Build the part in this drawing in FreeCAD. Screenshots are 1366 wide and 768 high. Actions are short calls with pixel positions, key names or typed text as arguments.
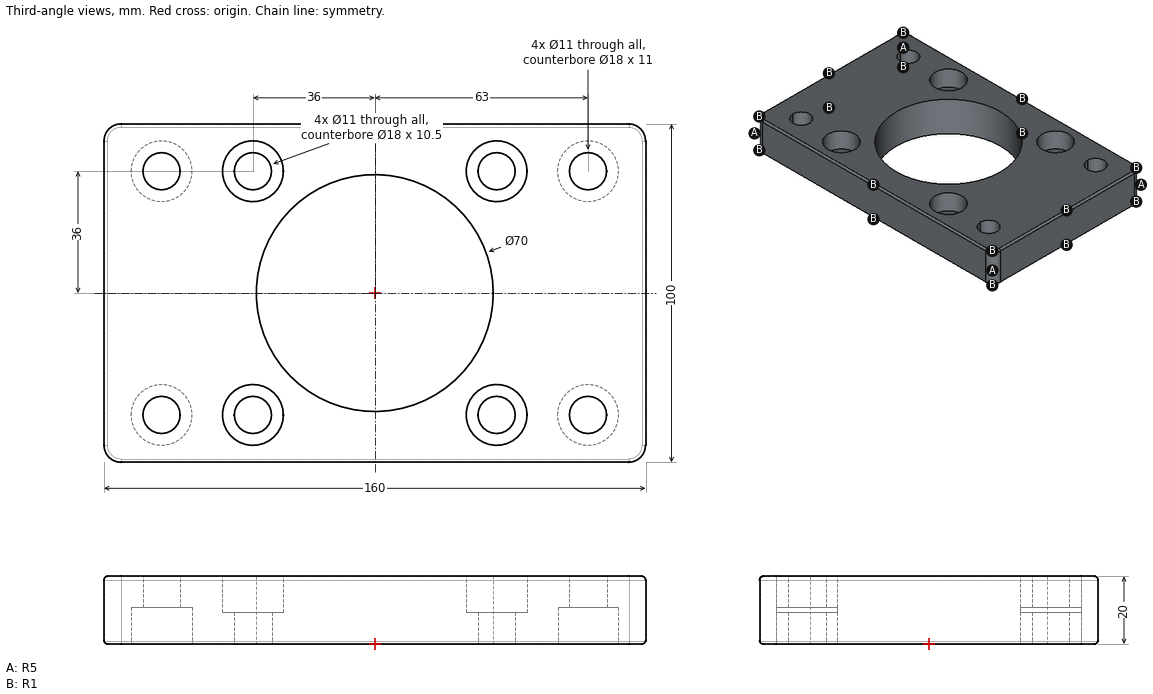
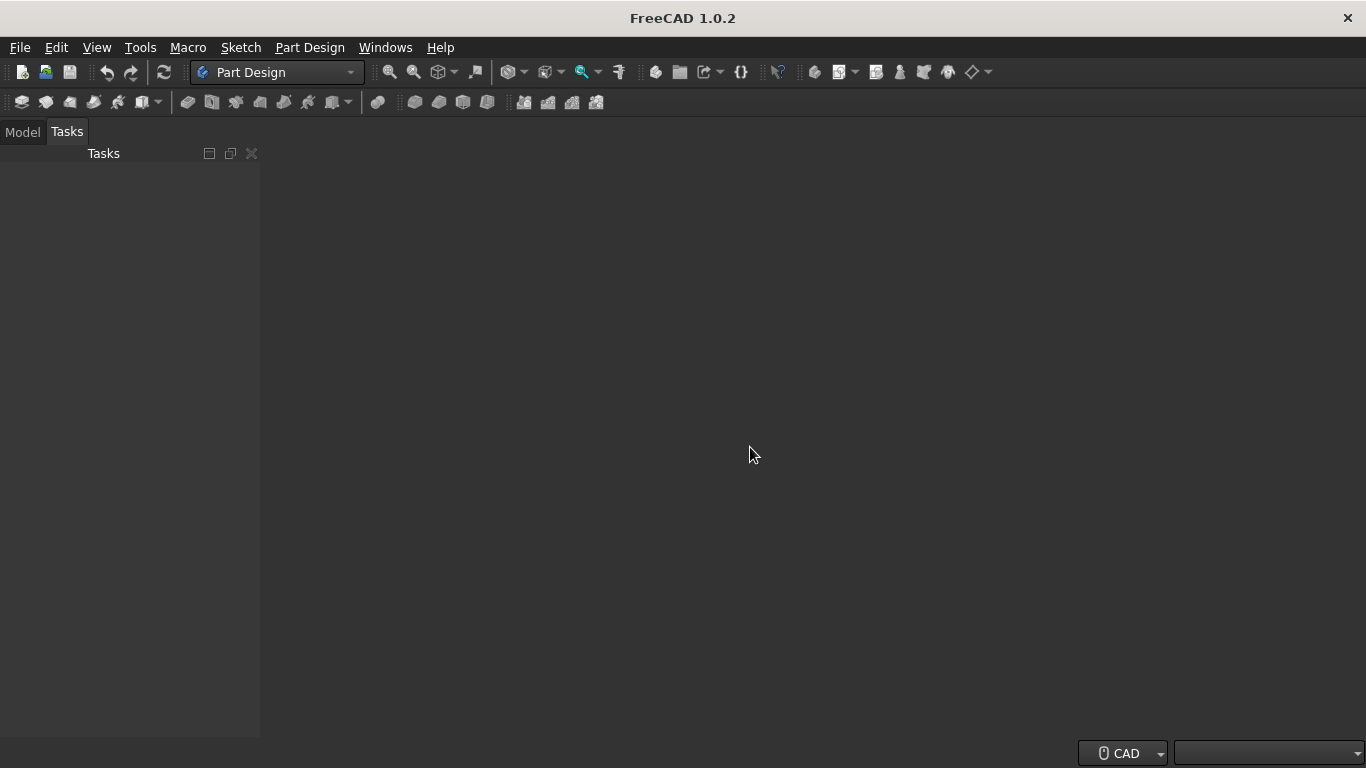
key(ctrl+n)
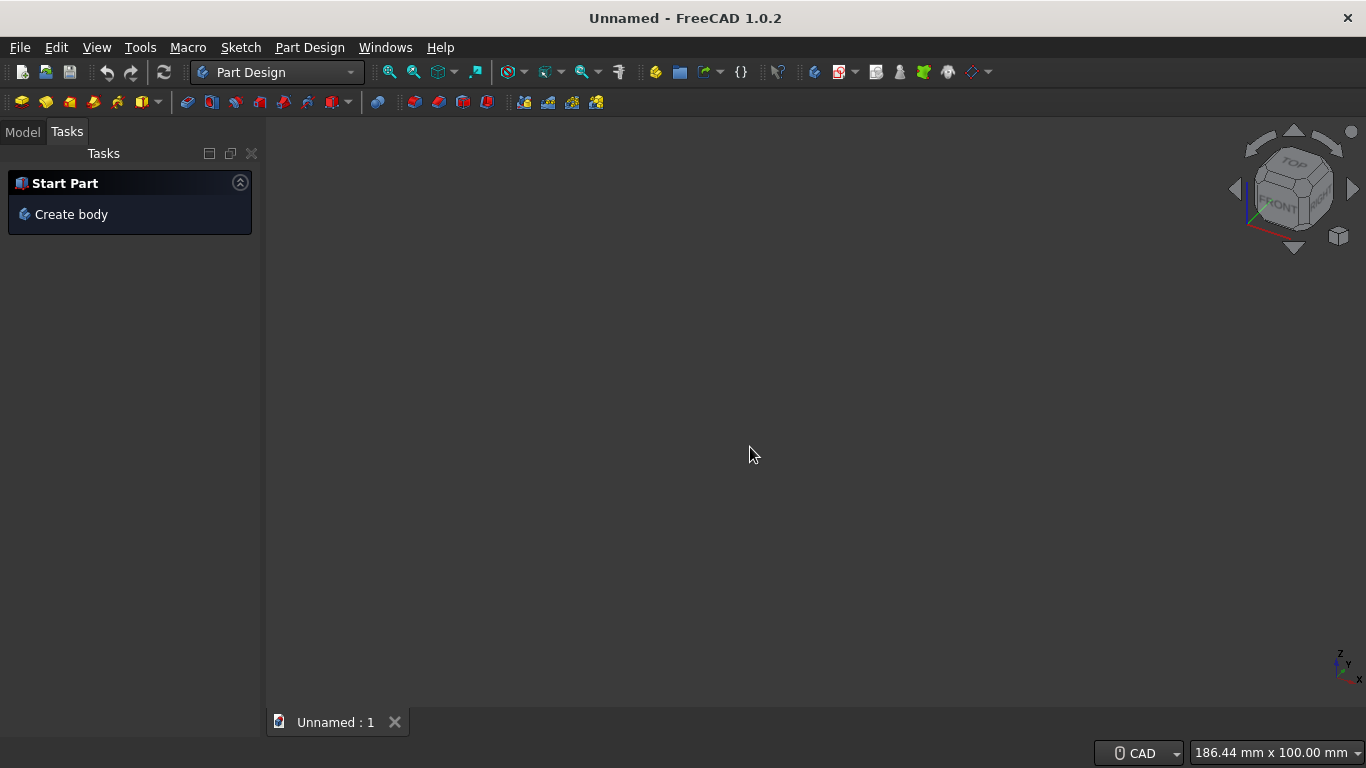
click(840, 72)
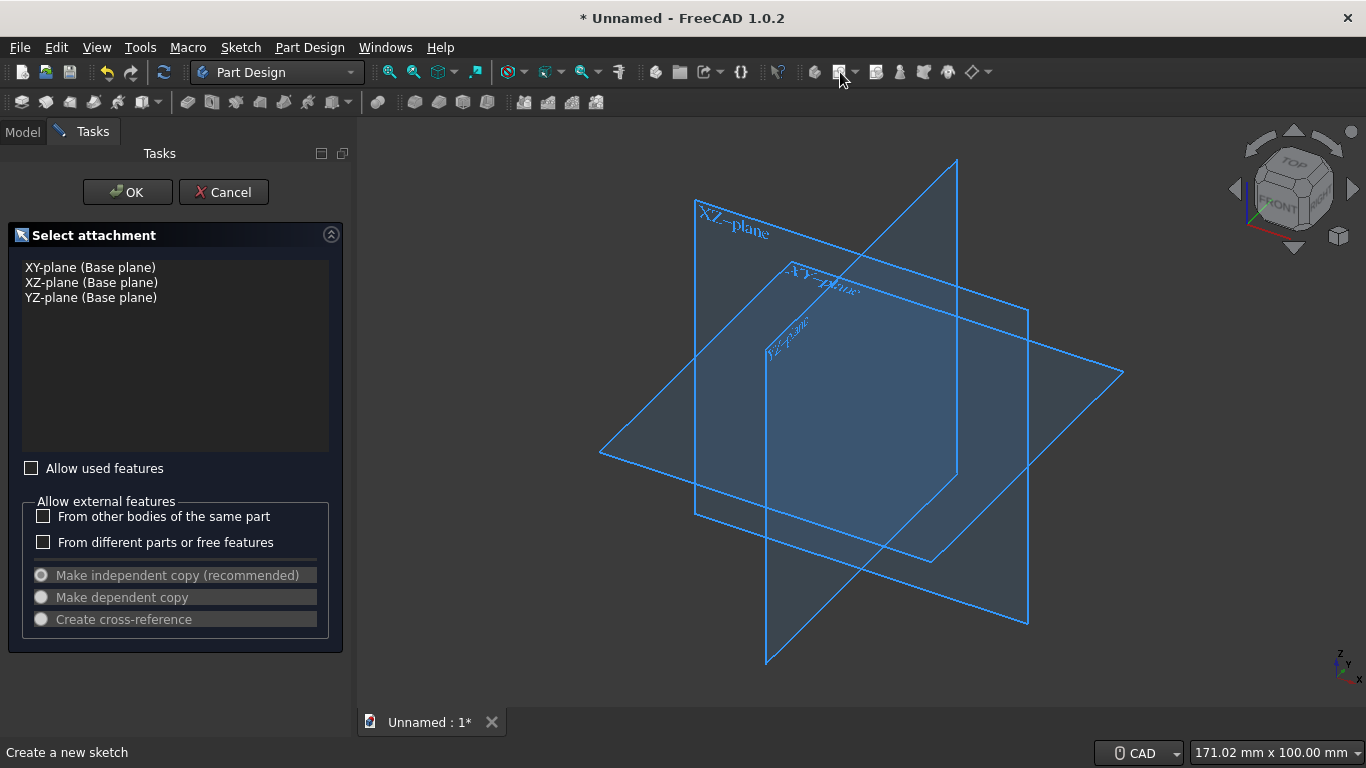
click(82, 268)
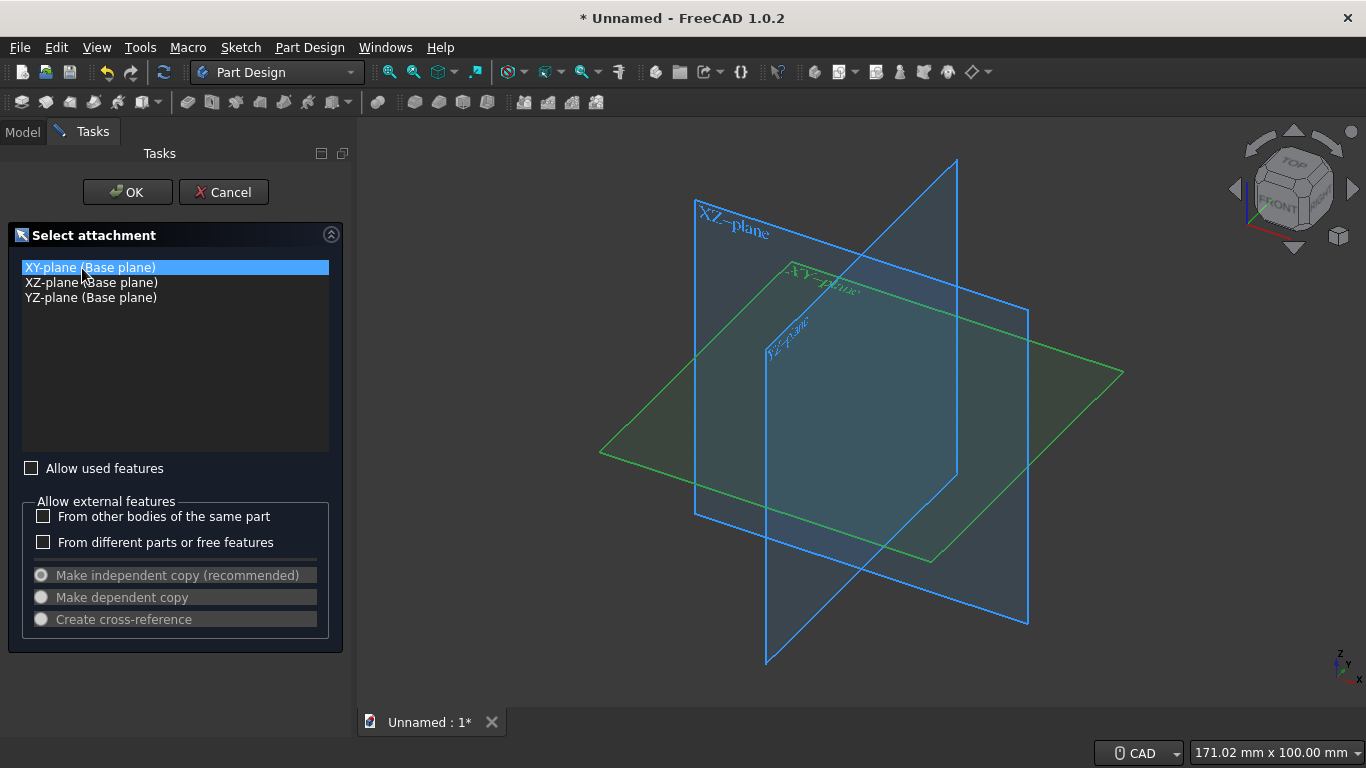
click(128, 192)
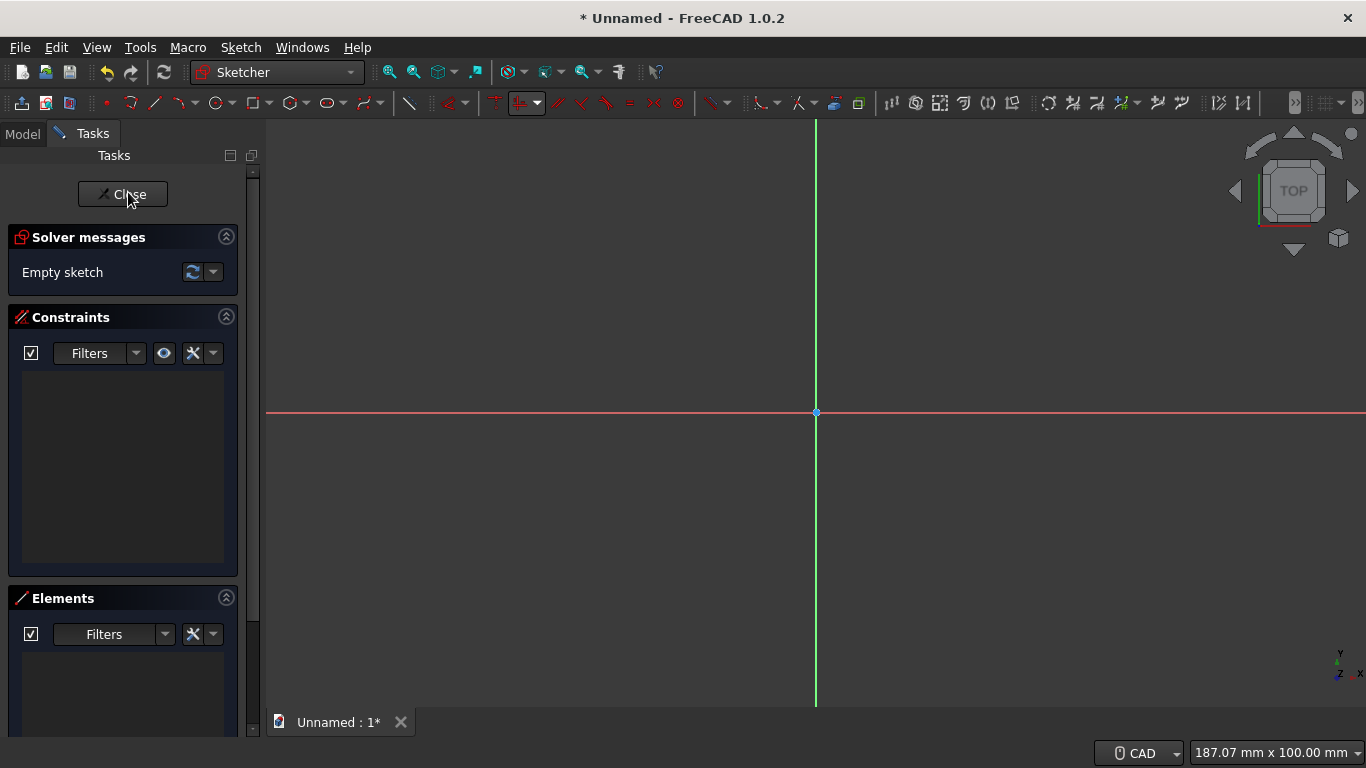
scroll(608, 413, down, 2)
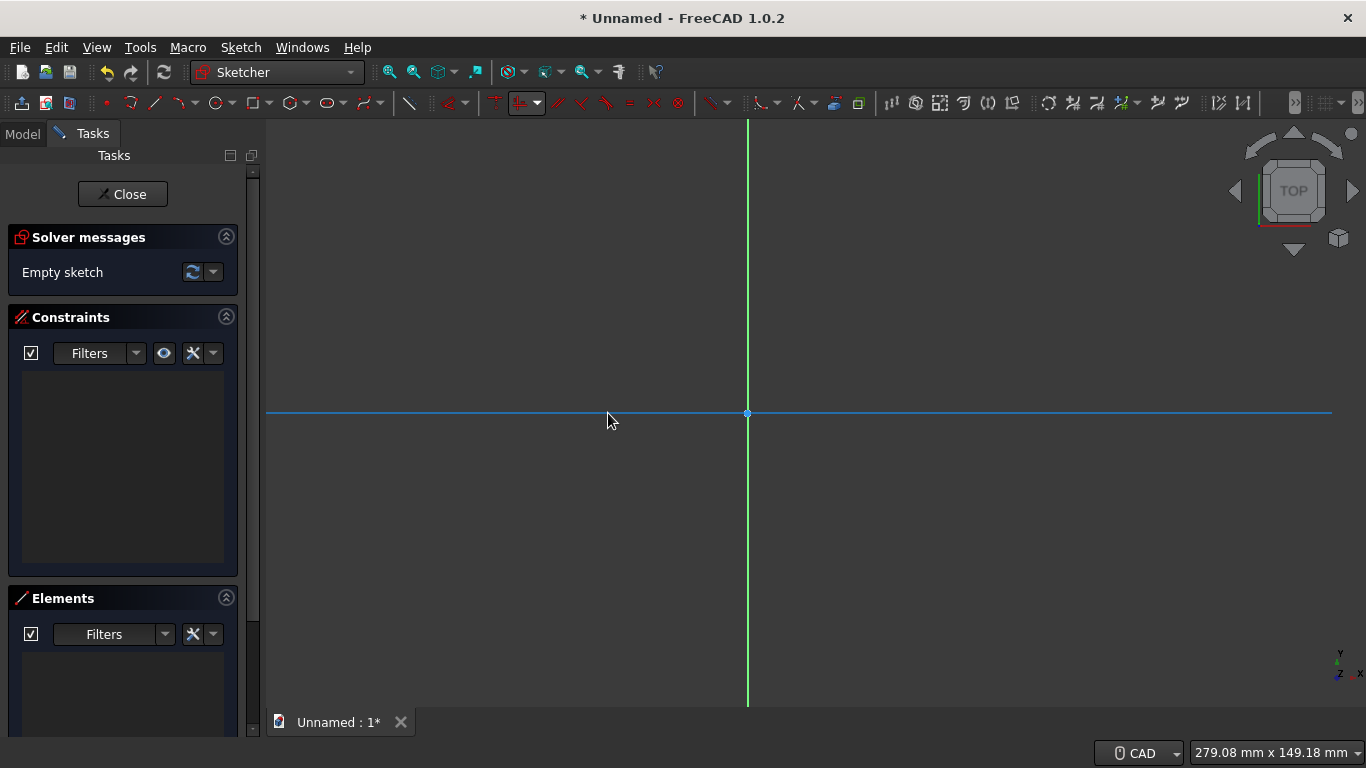
key(g)
key(v)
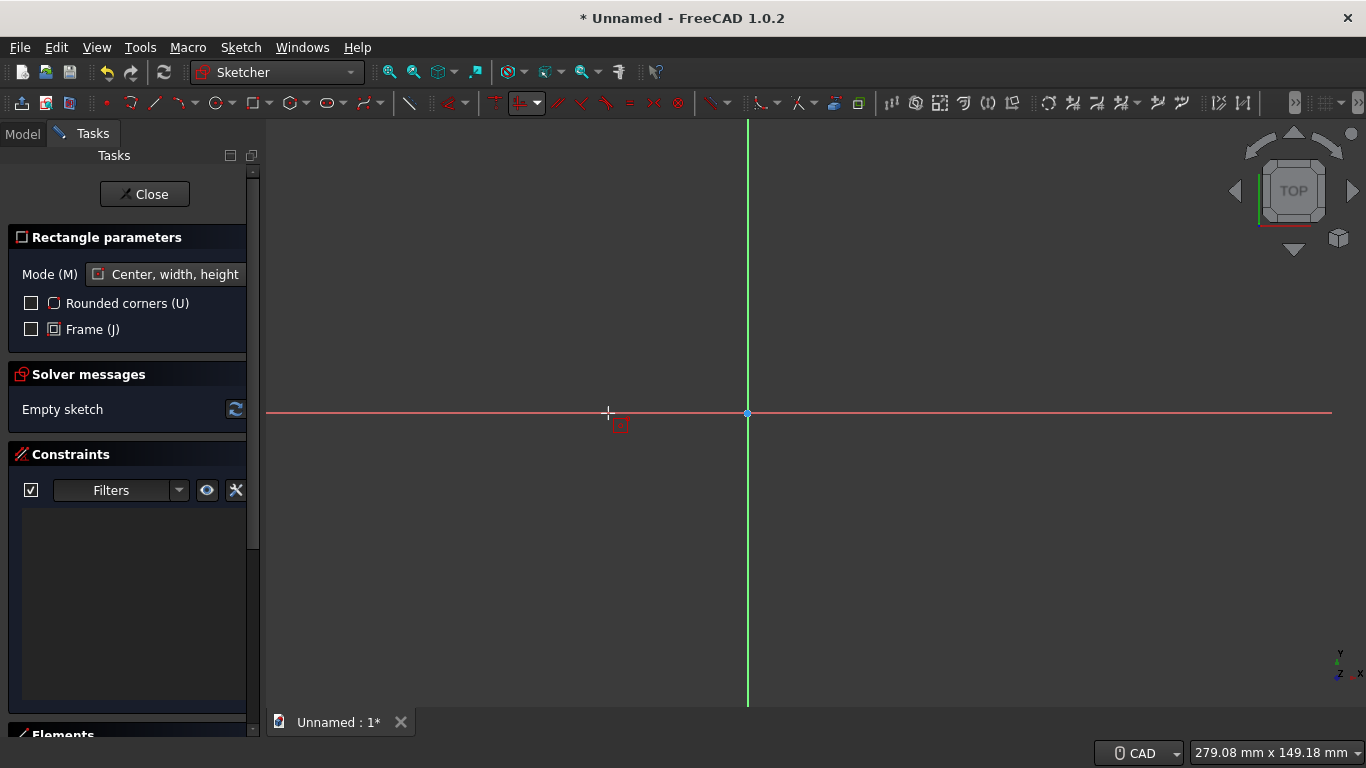
click(748, 413)
click(1063, 216)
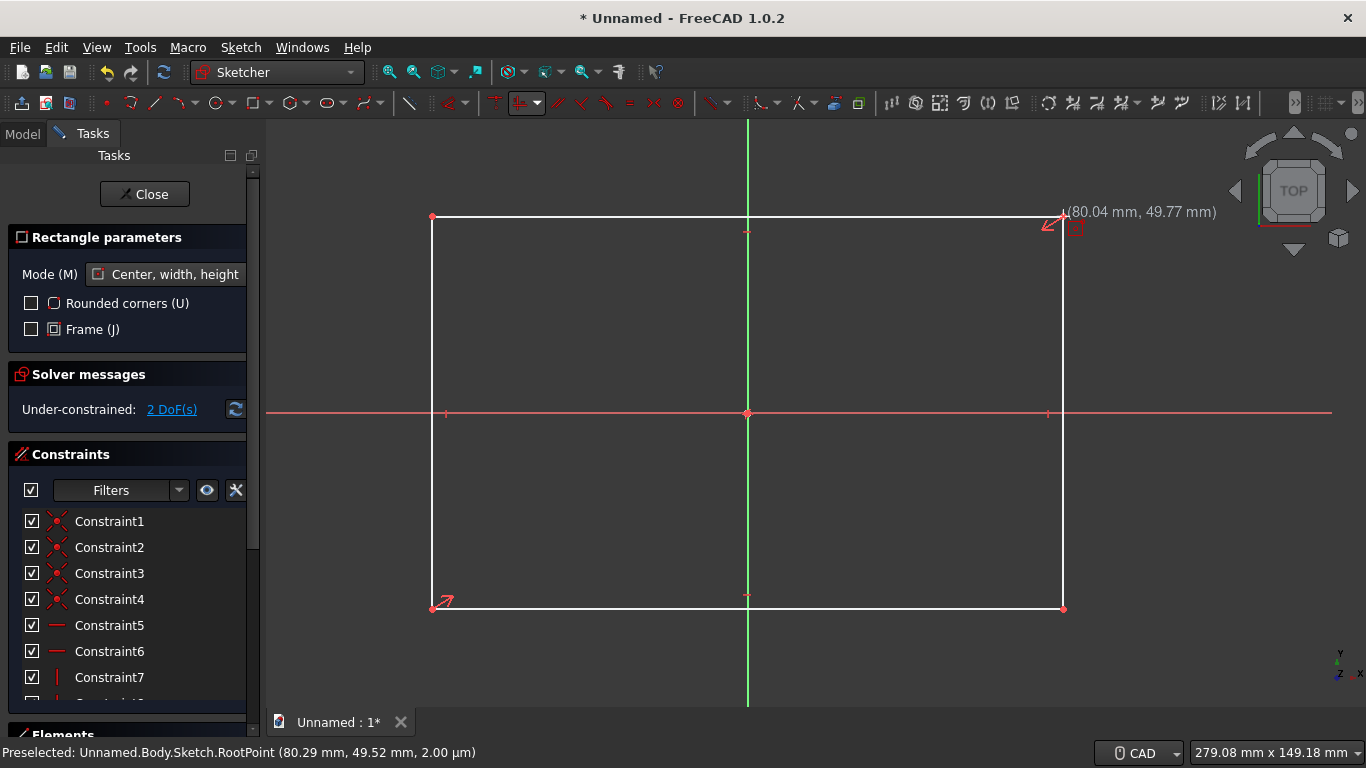
key(g)
key(c)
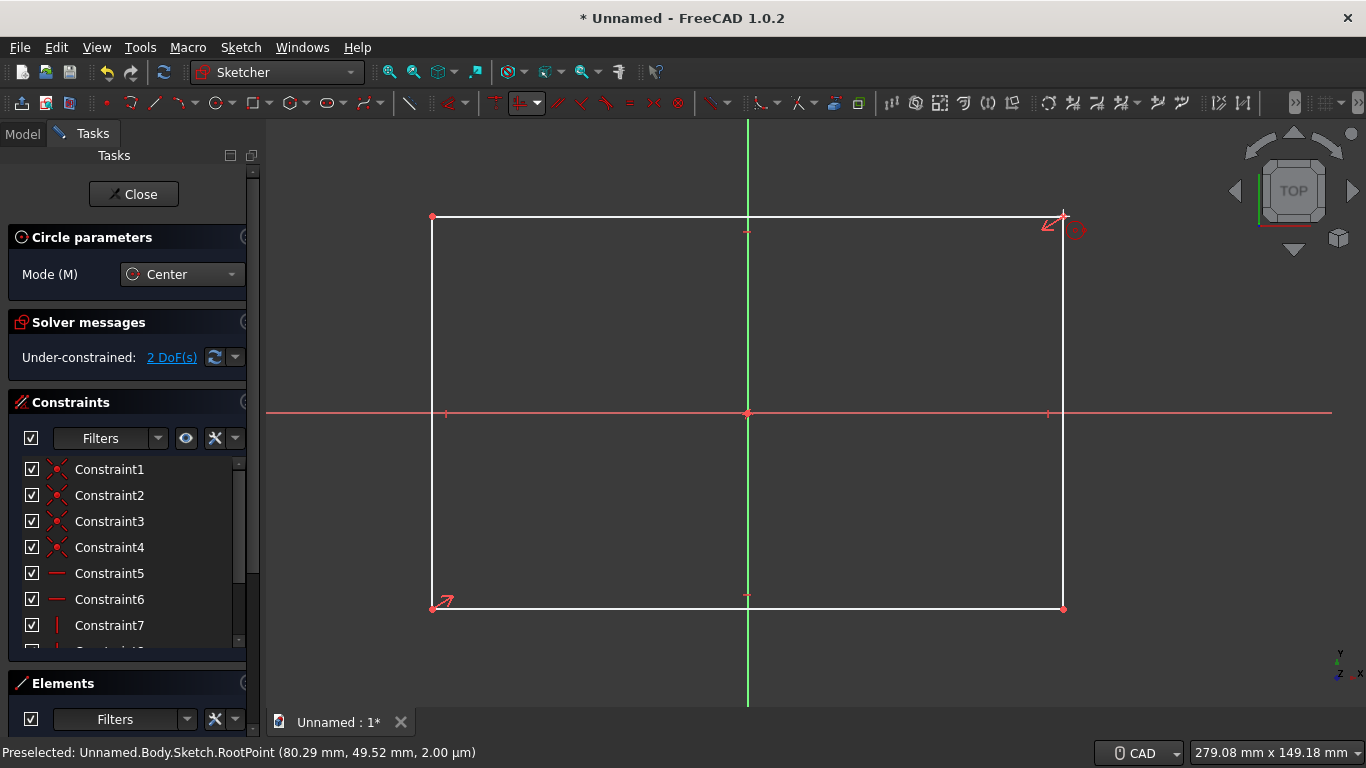
click(748, 413)
click(845, 316)
key(Escape)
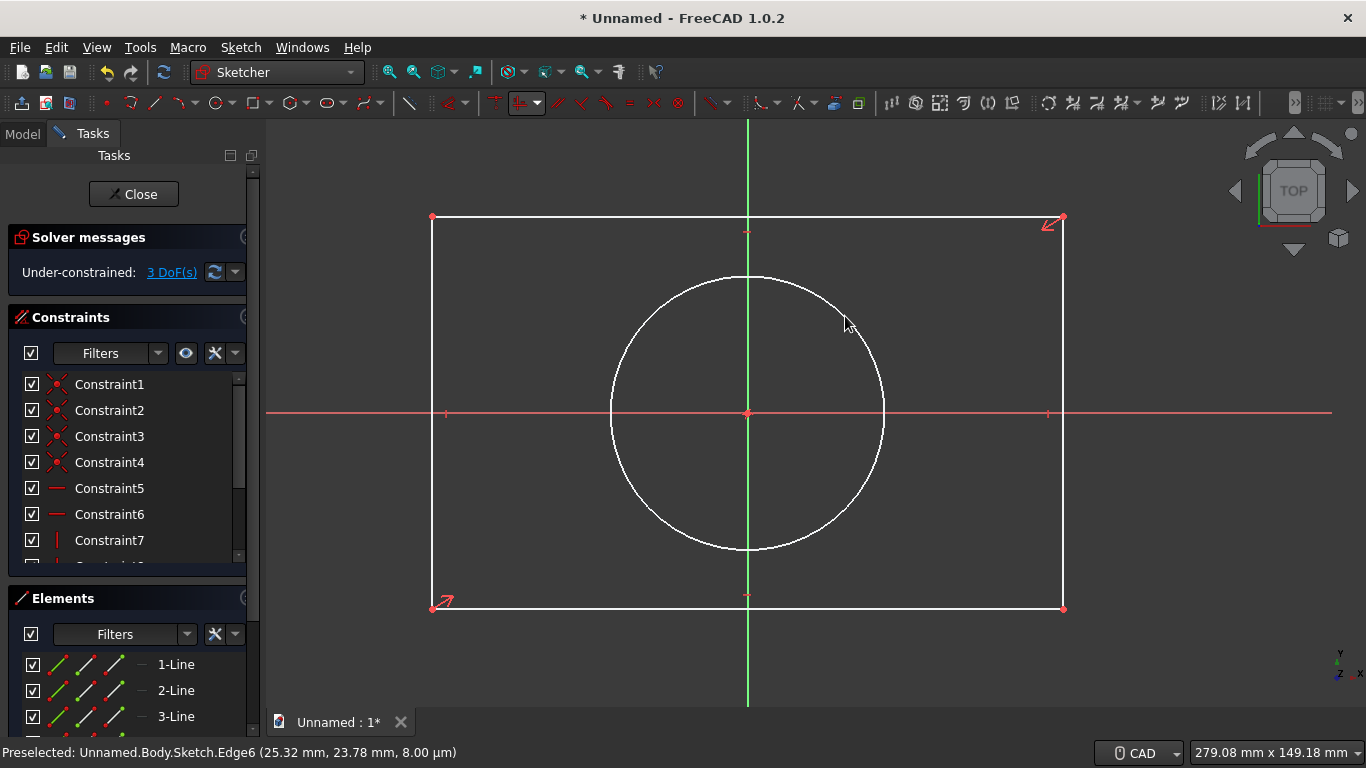
key(d)